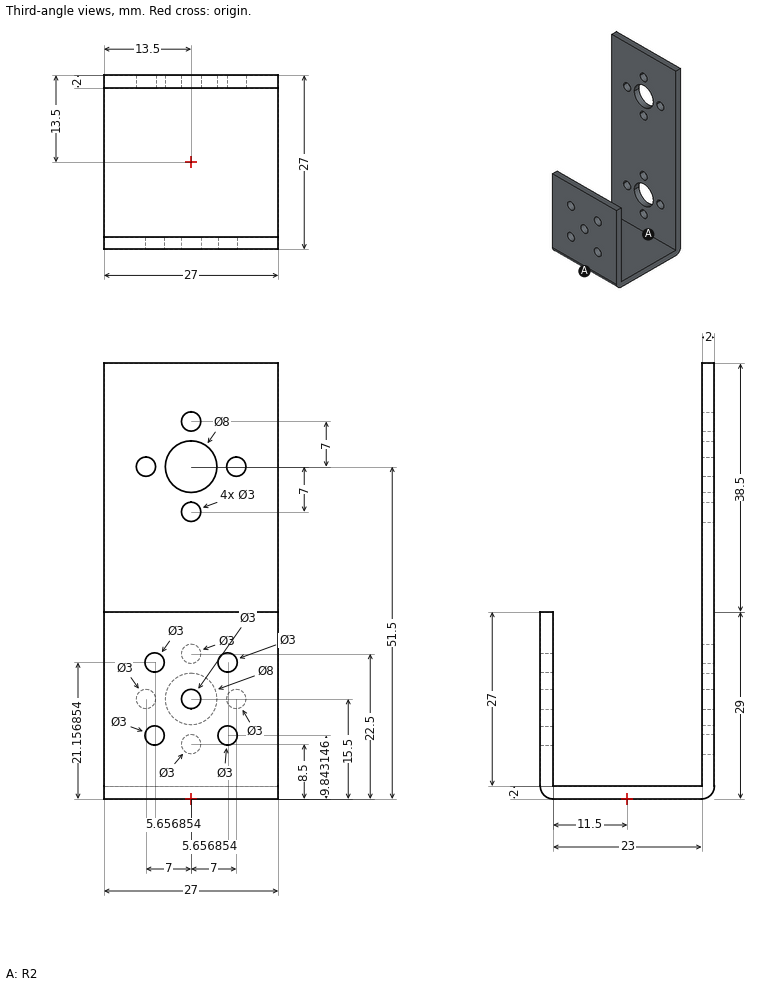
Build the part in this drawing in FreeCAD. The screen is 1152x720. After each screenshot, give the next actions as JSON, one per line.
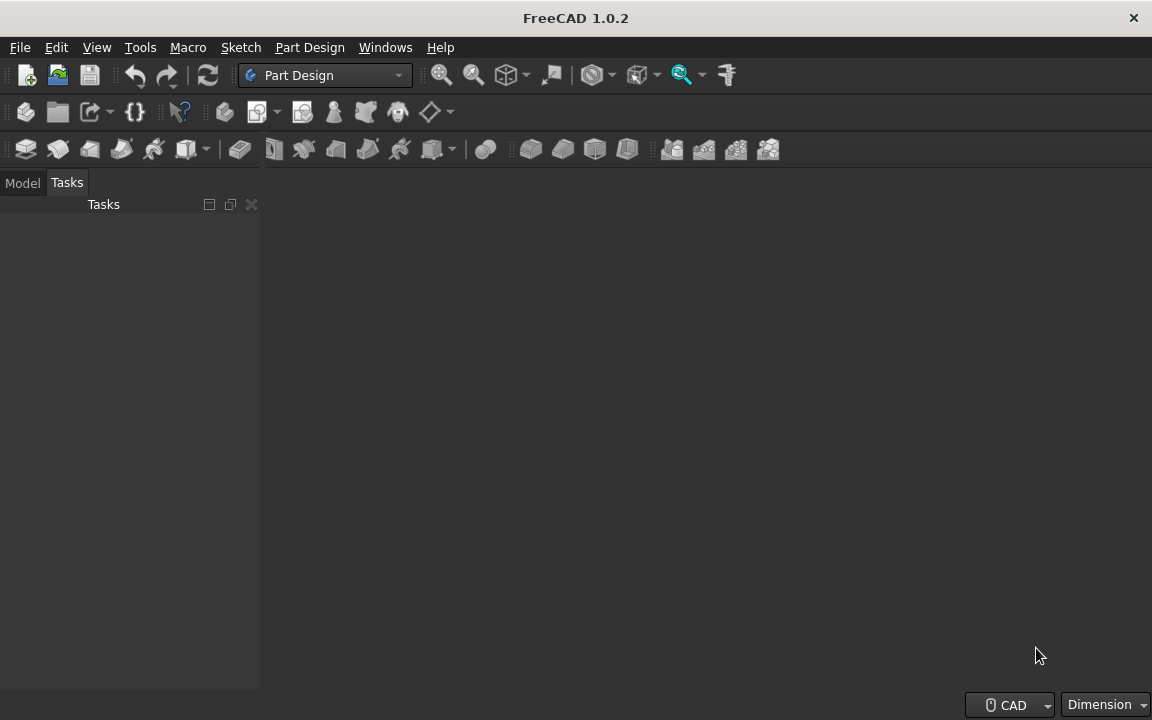
{"action": "key", "text": "ctrl+n"}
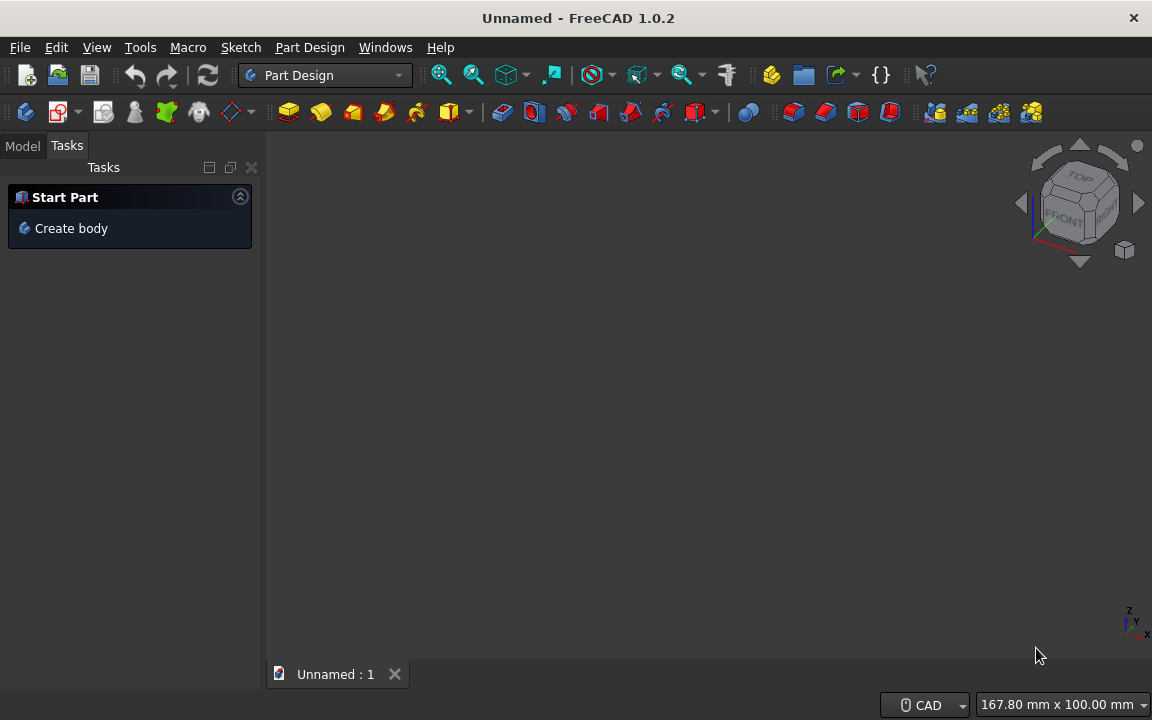
{"action": "left_click", "coordinate": [58, 112]}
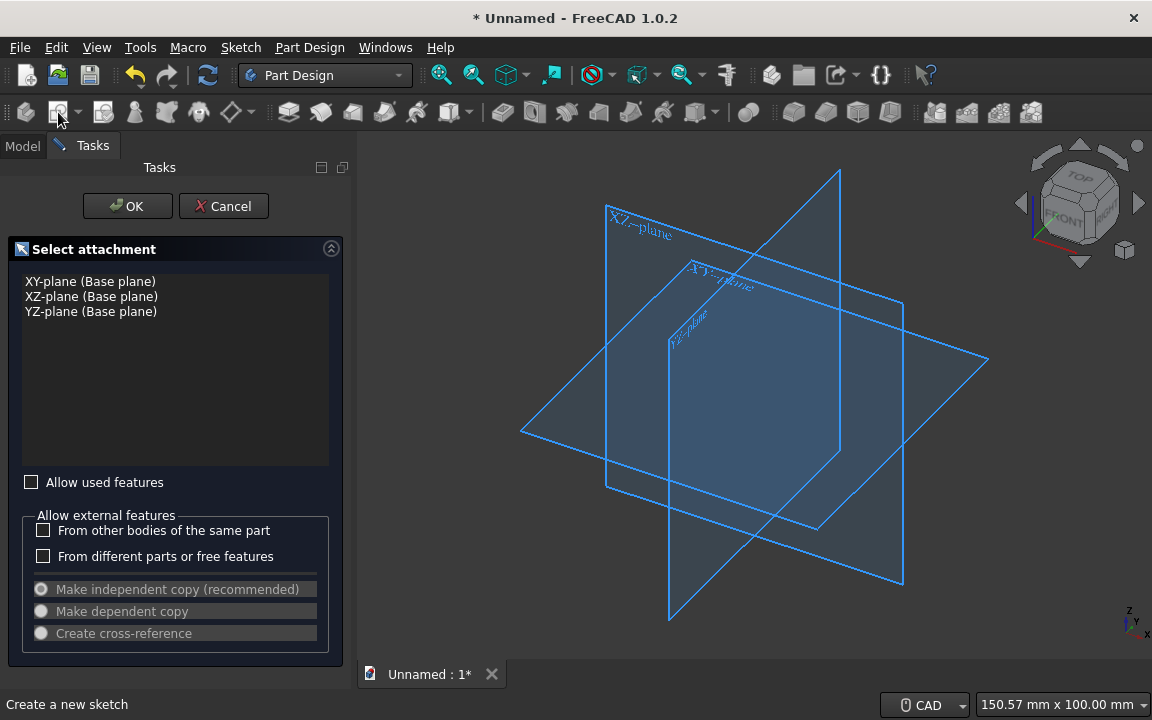
{"action": "left_click", "coordinate": [82, 282]}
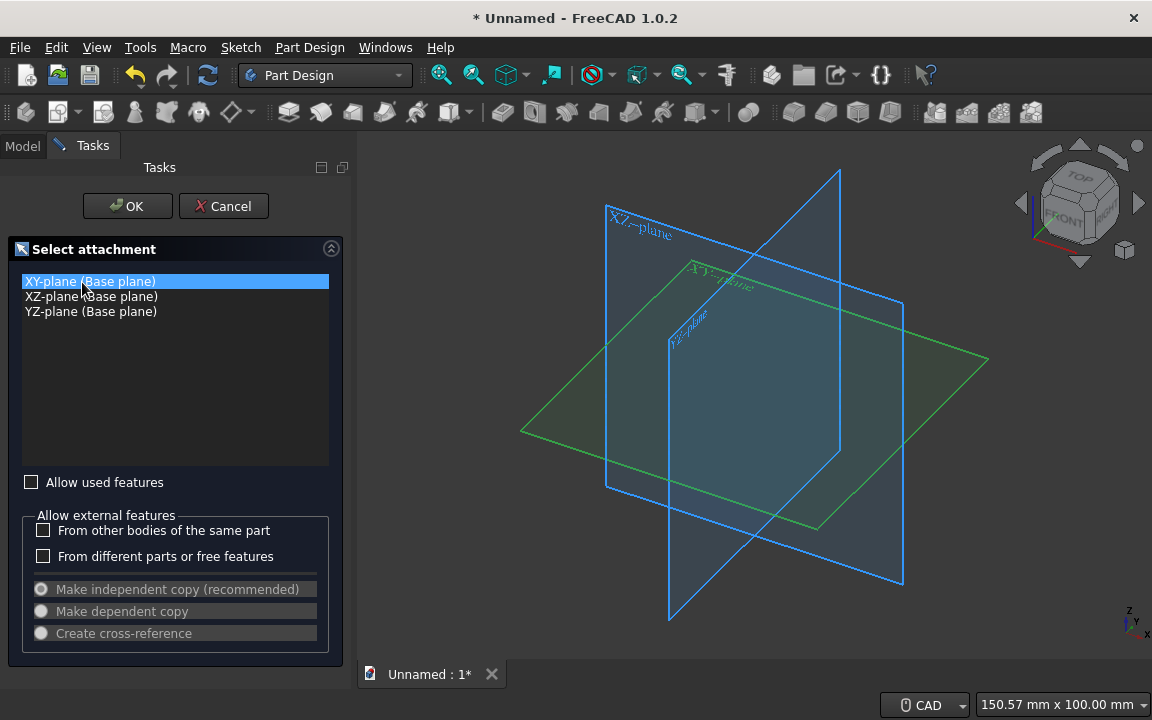
{"action": "left_click", "coordinate": [128, 206]}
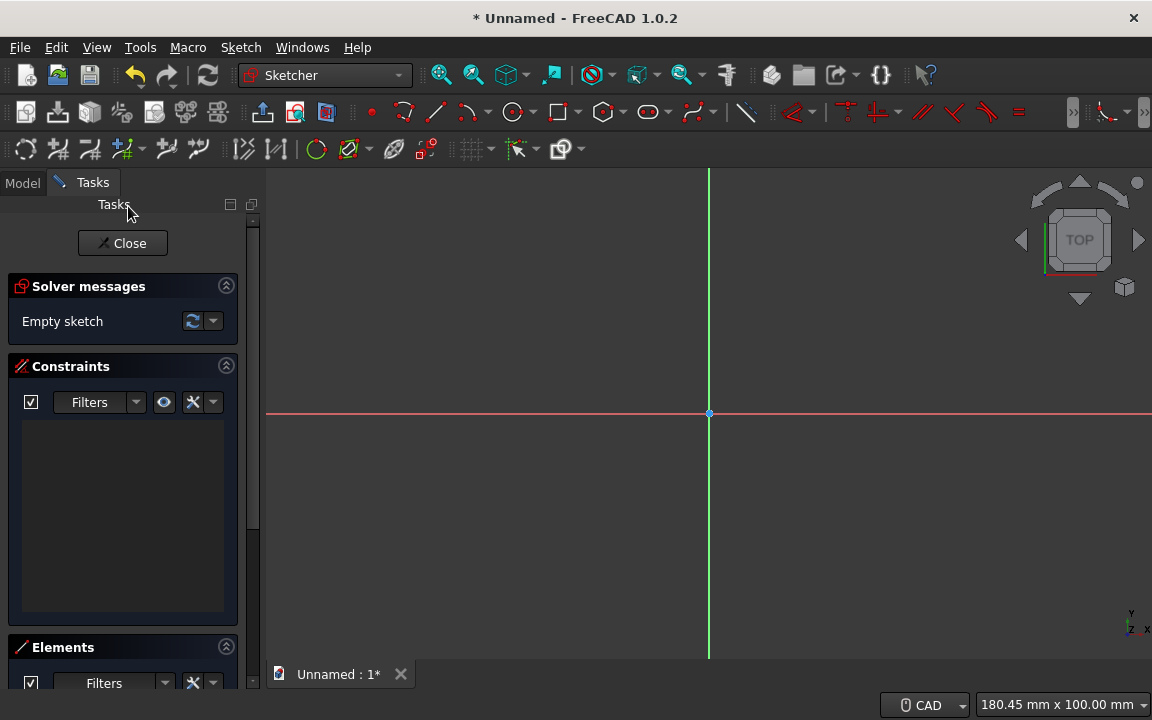
{"action": "scroll", "coordinate": [765, 413], "scroll_direction": "up", "scroll_amount": 4}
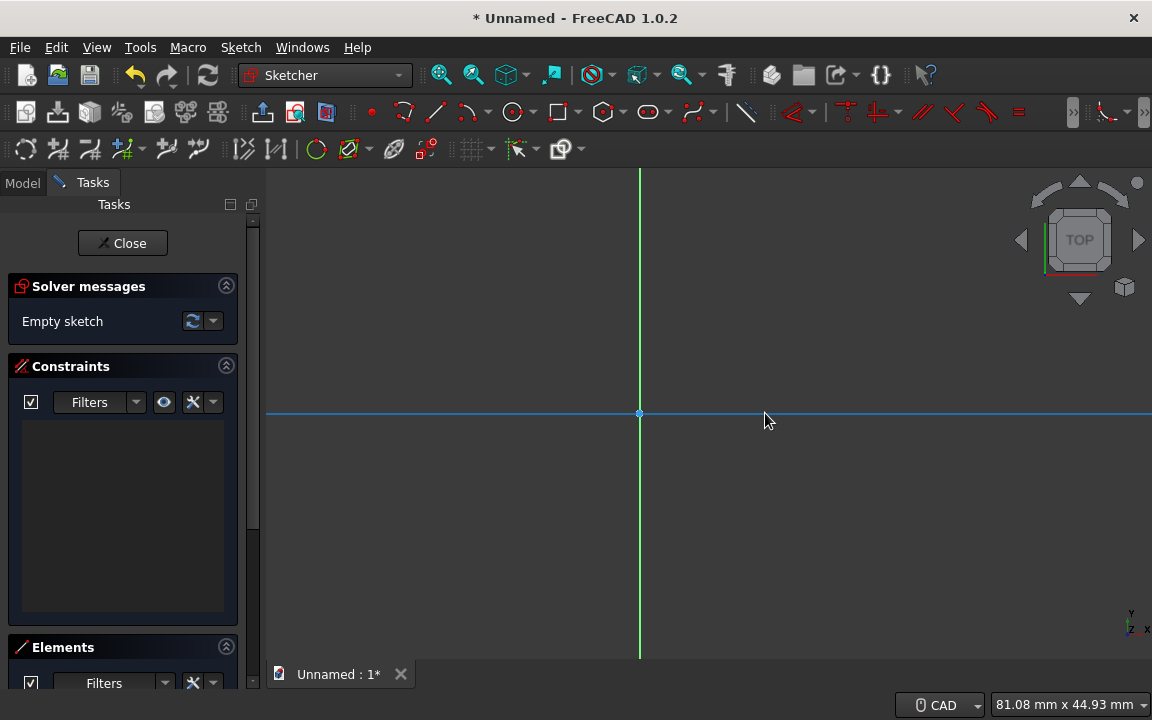
{"action": "key", "text": "g v"}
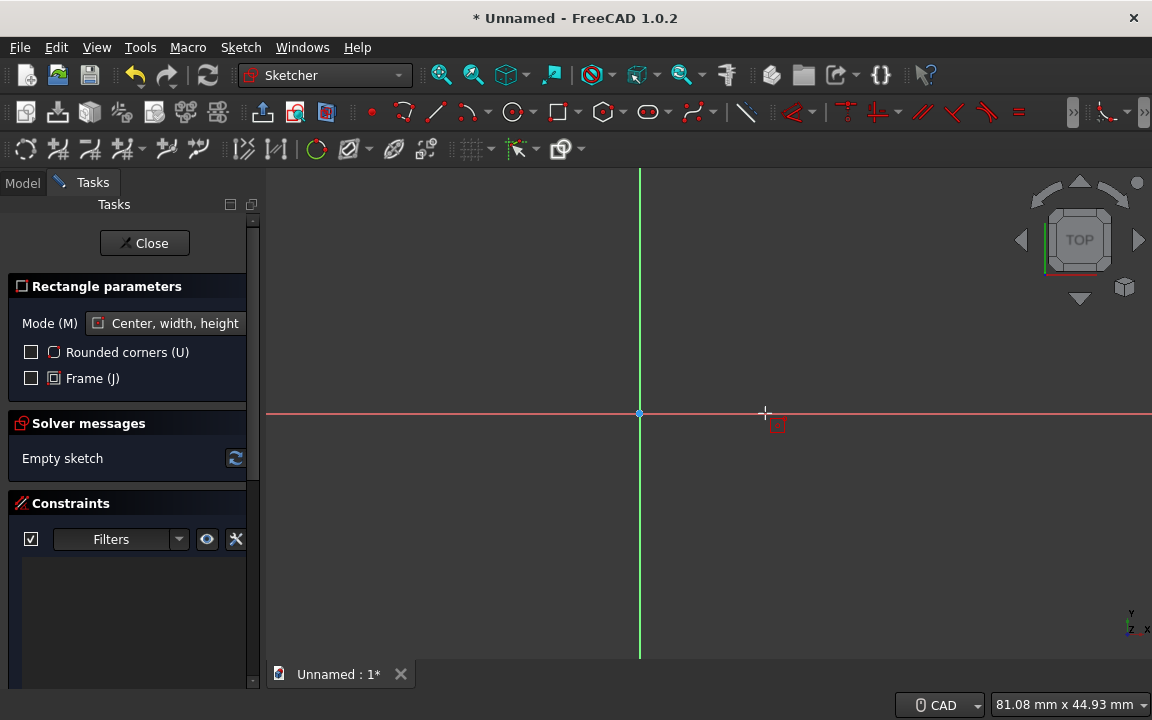
{"action": "left_click", "coordinate": [640, 414]}
{"action": "left_click", "coordinate": [787, 266]}
{"action": "key", "text": "Escape"}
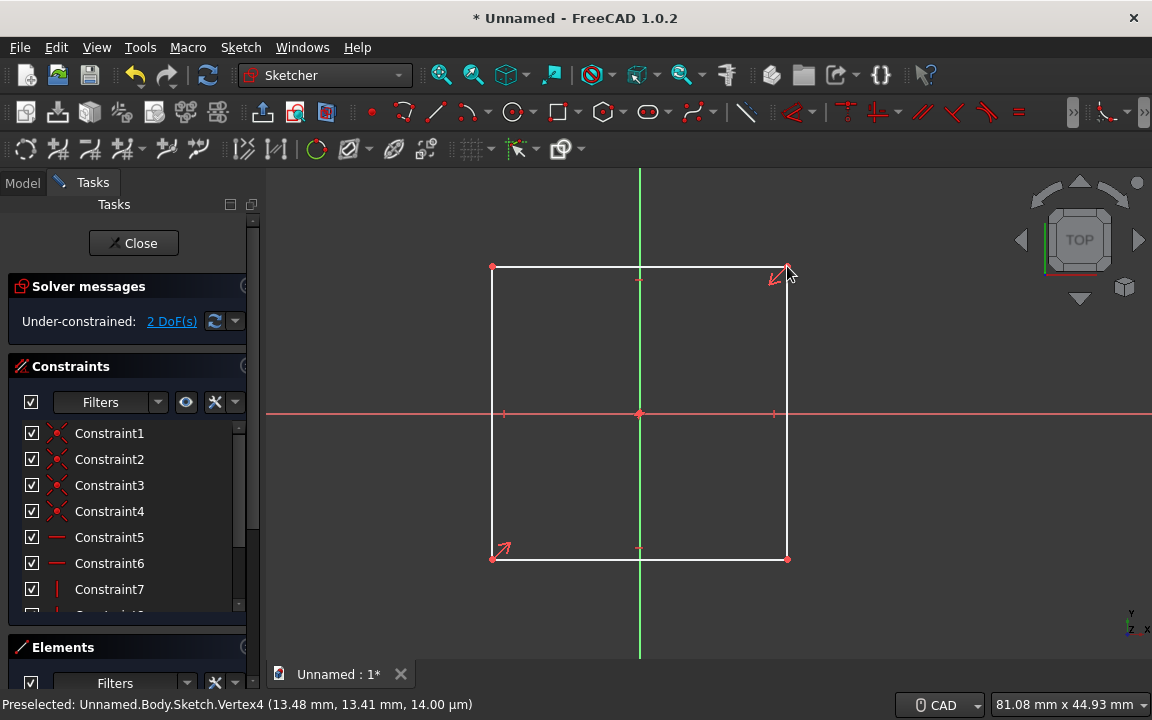
{"action": "key", "text": "d"}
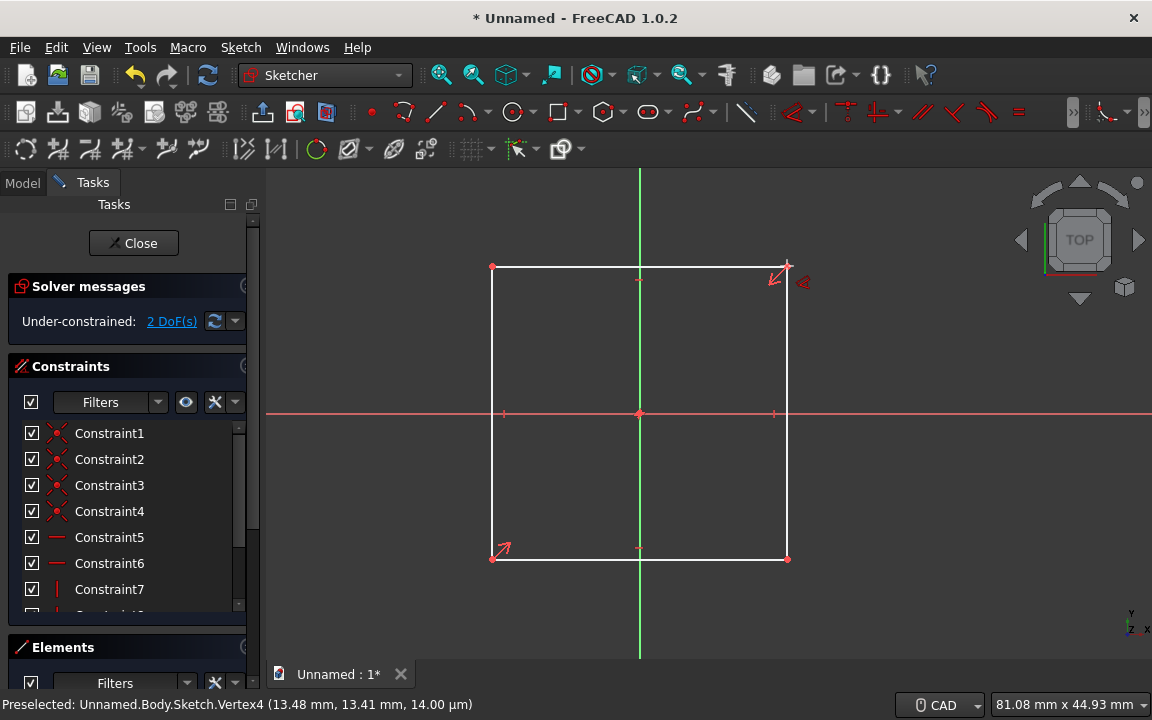
{"action": "left_click", "coordinate": [581, 560]}
{"action": "left_click", "coordinate": [572, 594]}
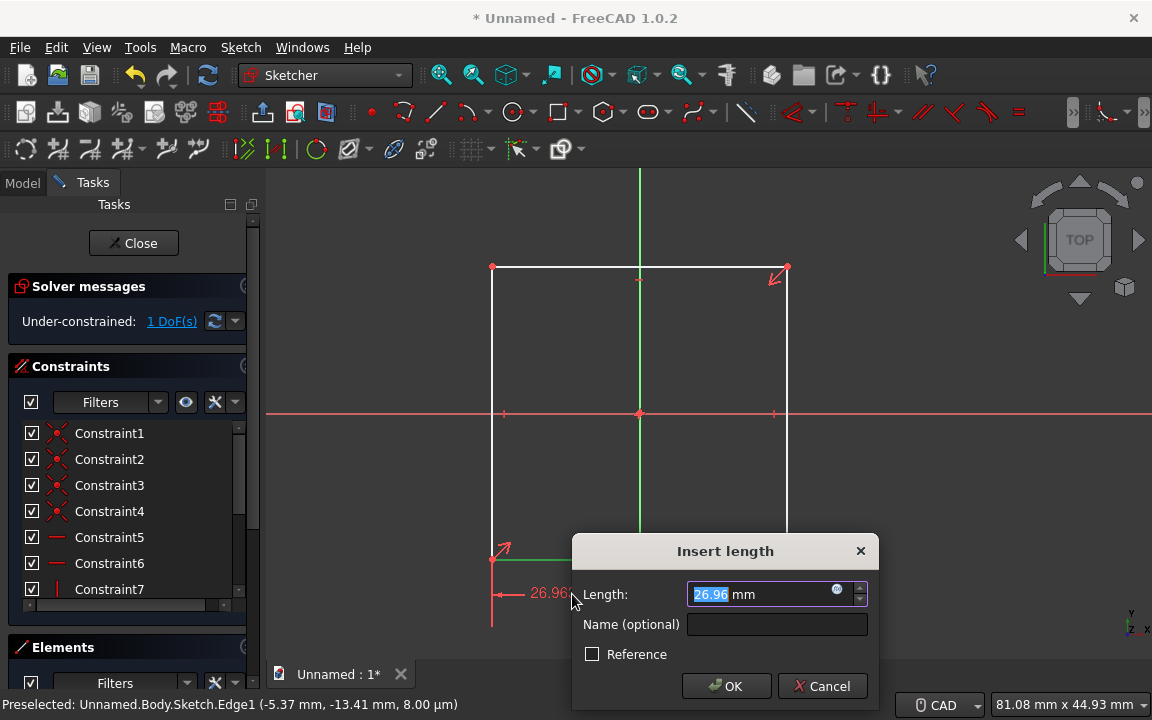
{"action": "type", "text": "27"}
{"action": "key", "text": "Return"}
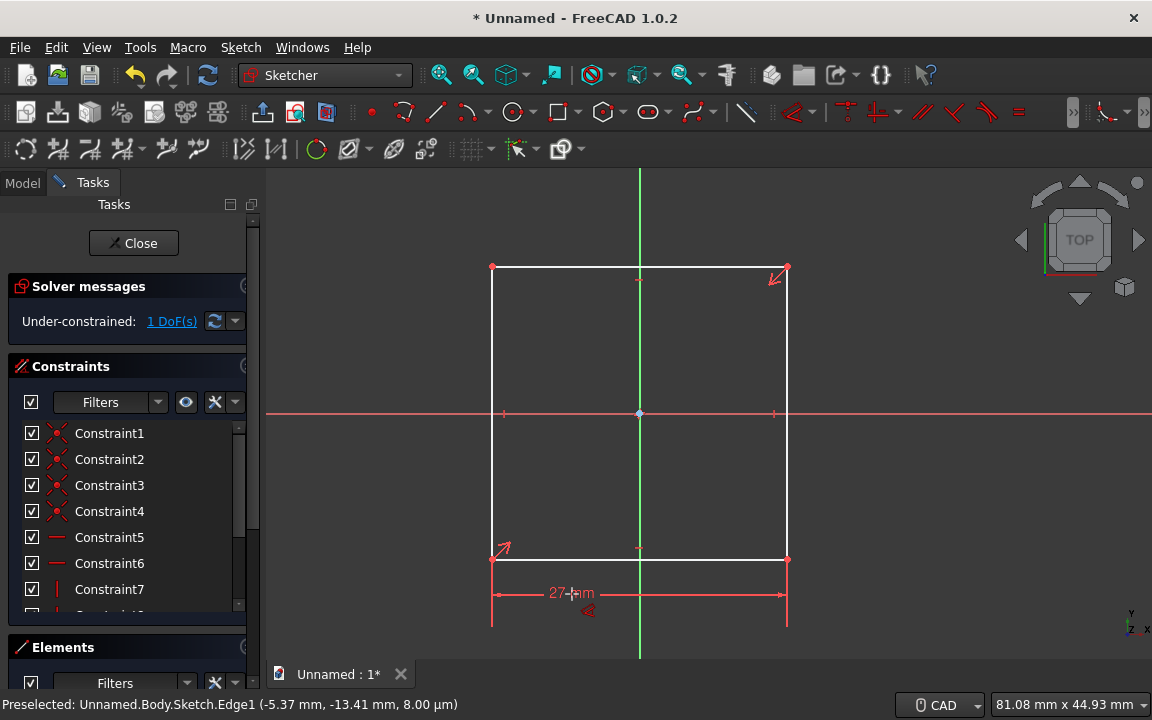
{"action": "left_click", "coordinate": [787, 472]}
{"action": "left_click", "coordinate": [821, 346]}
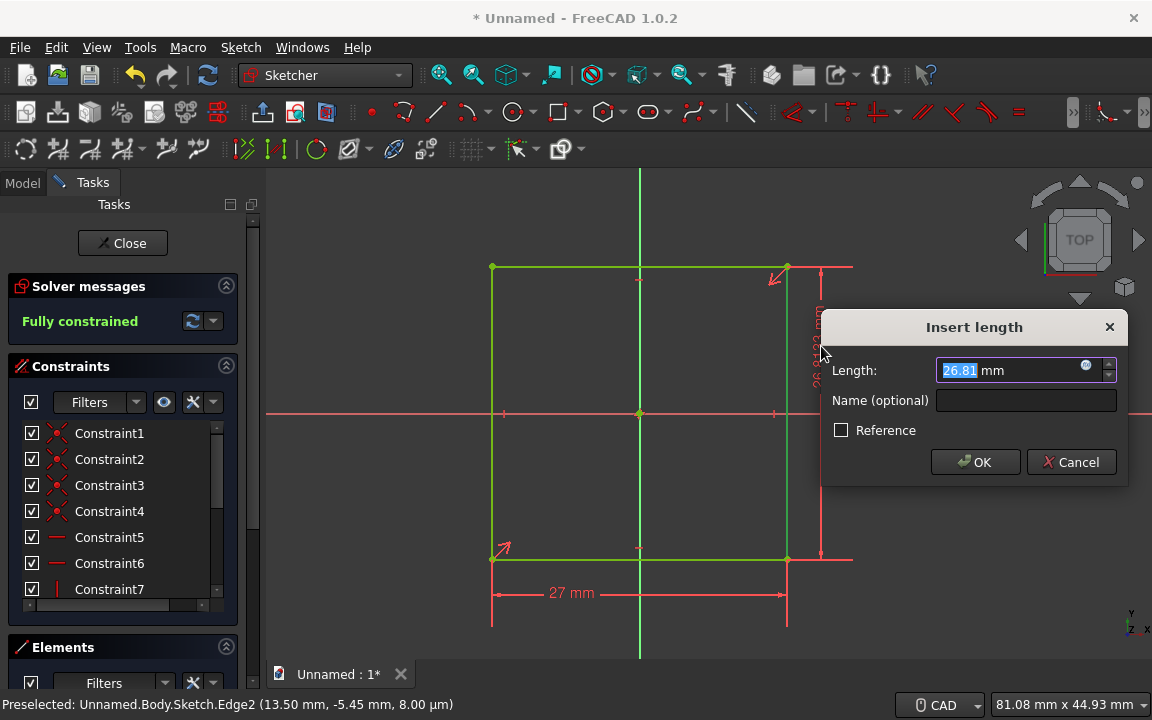
{"action": "type", "text": "27"}
{"action": "key", "text": "Return"}
{"action": "key", "text": "Escape"}